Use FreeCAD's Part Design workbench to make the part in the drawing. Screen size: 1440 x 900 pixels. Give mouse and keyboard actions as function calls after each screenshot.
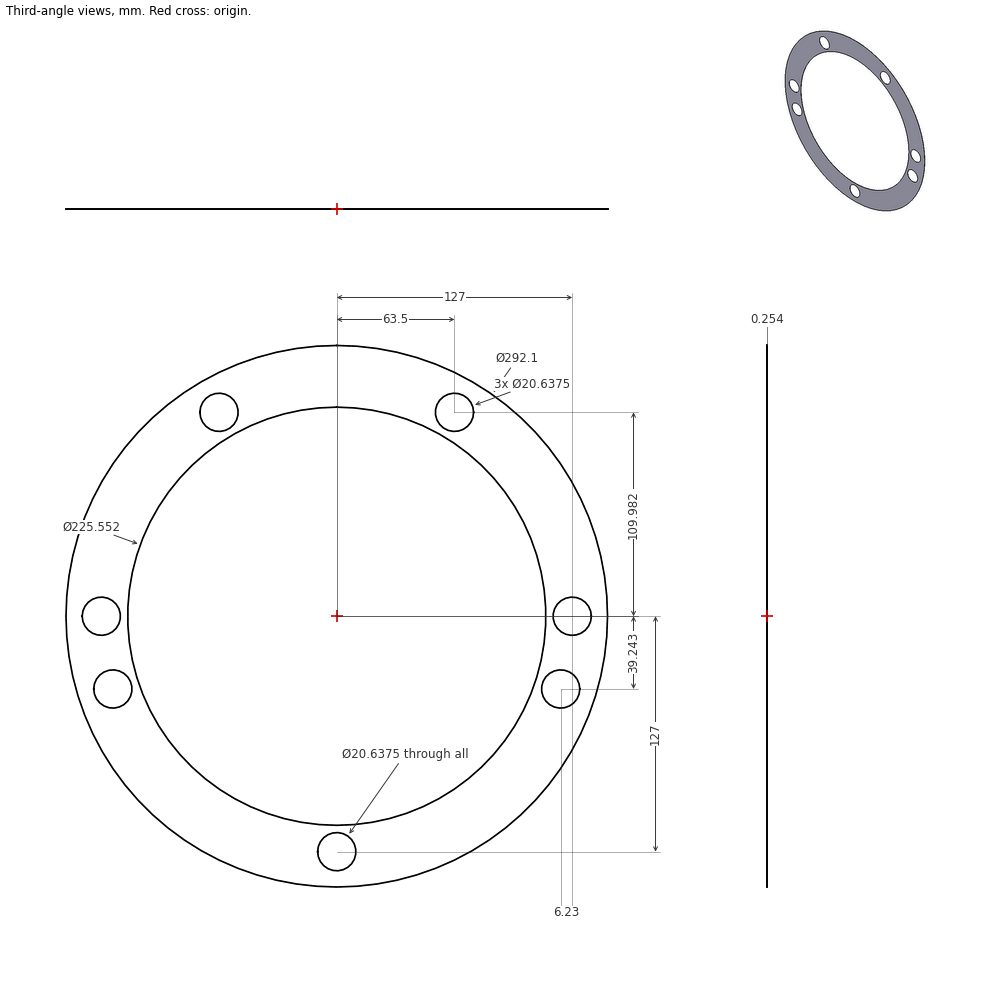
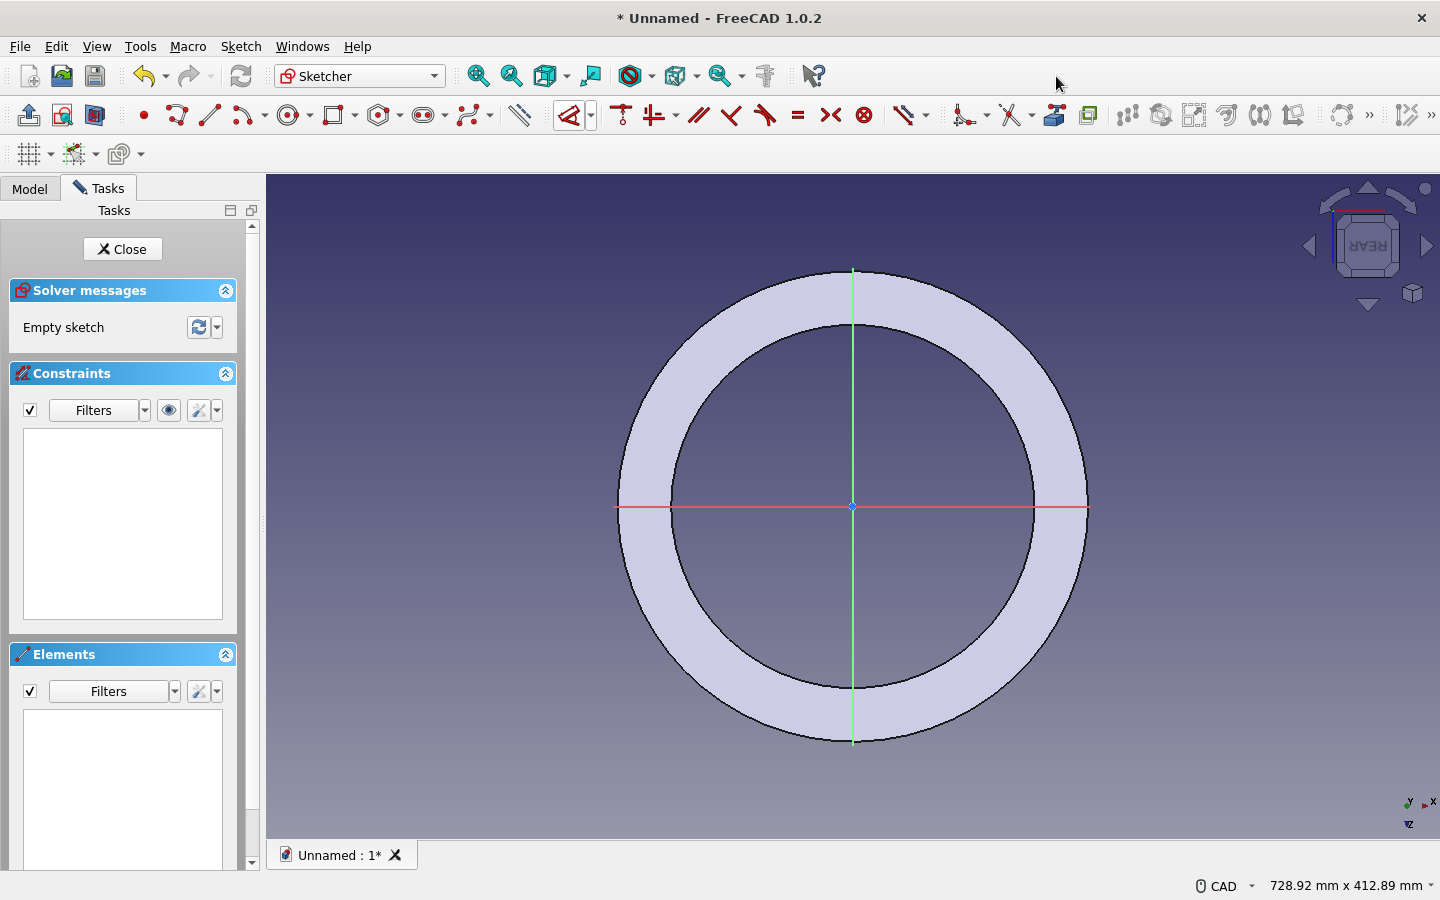
scroll(858, 286, up, 13)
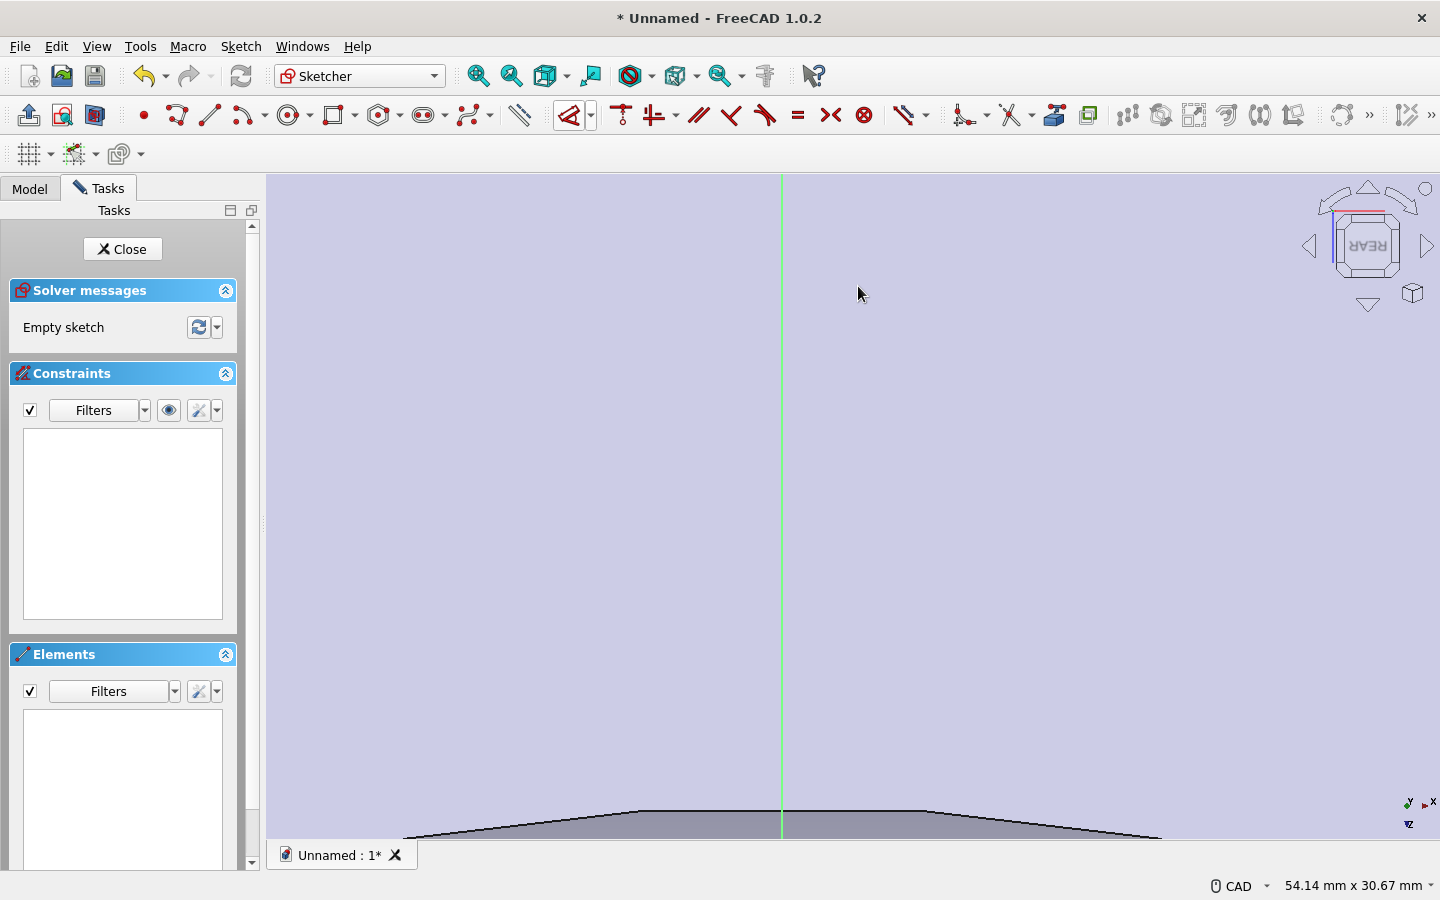
key(g)
key(c)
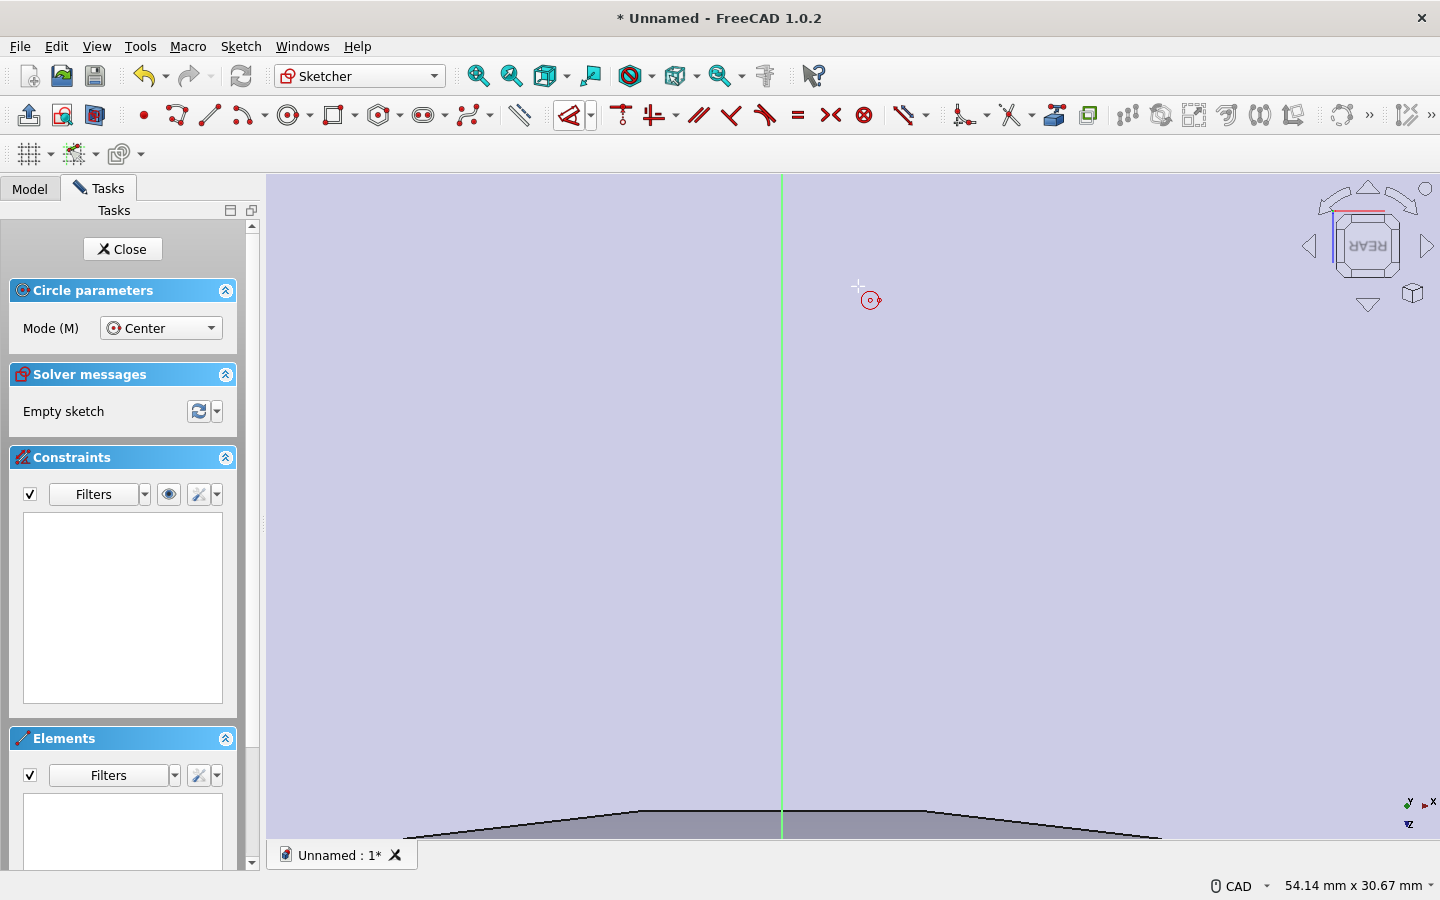
click(782, 499)
click(941, 340)
key(Escape)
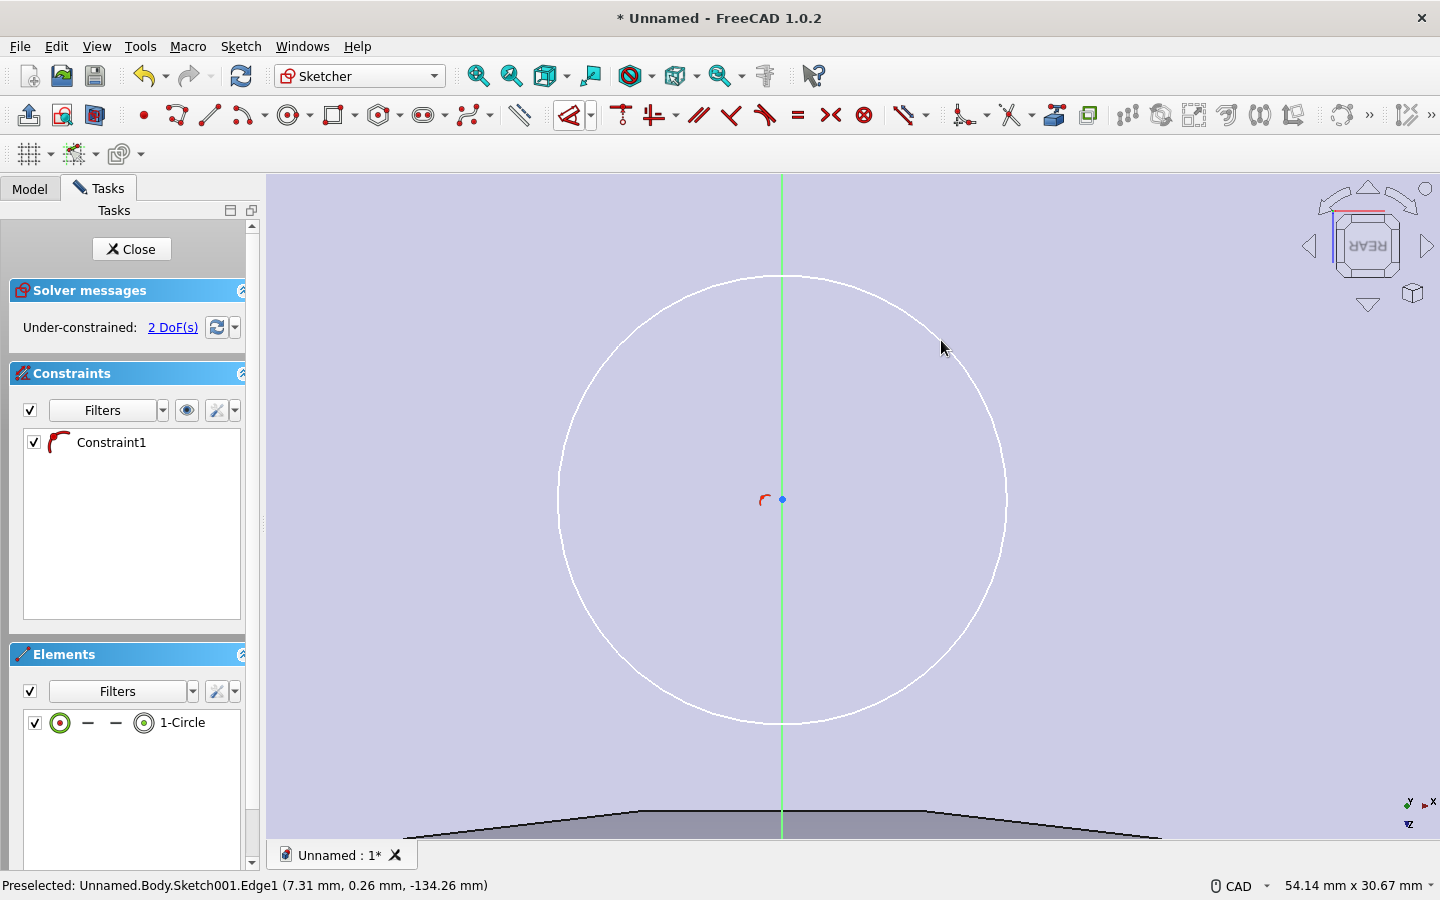
click(941, 341)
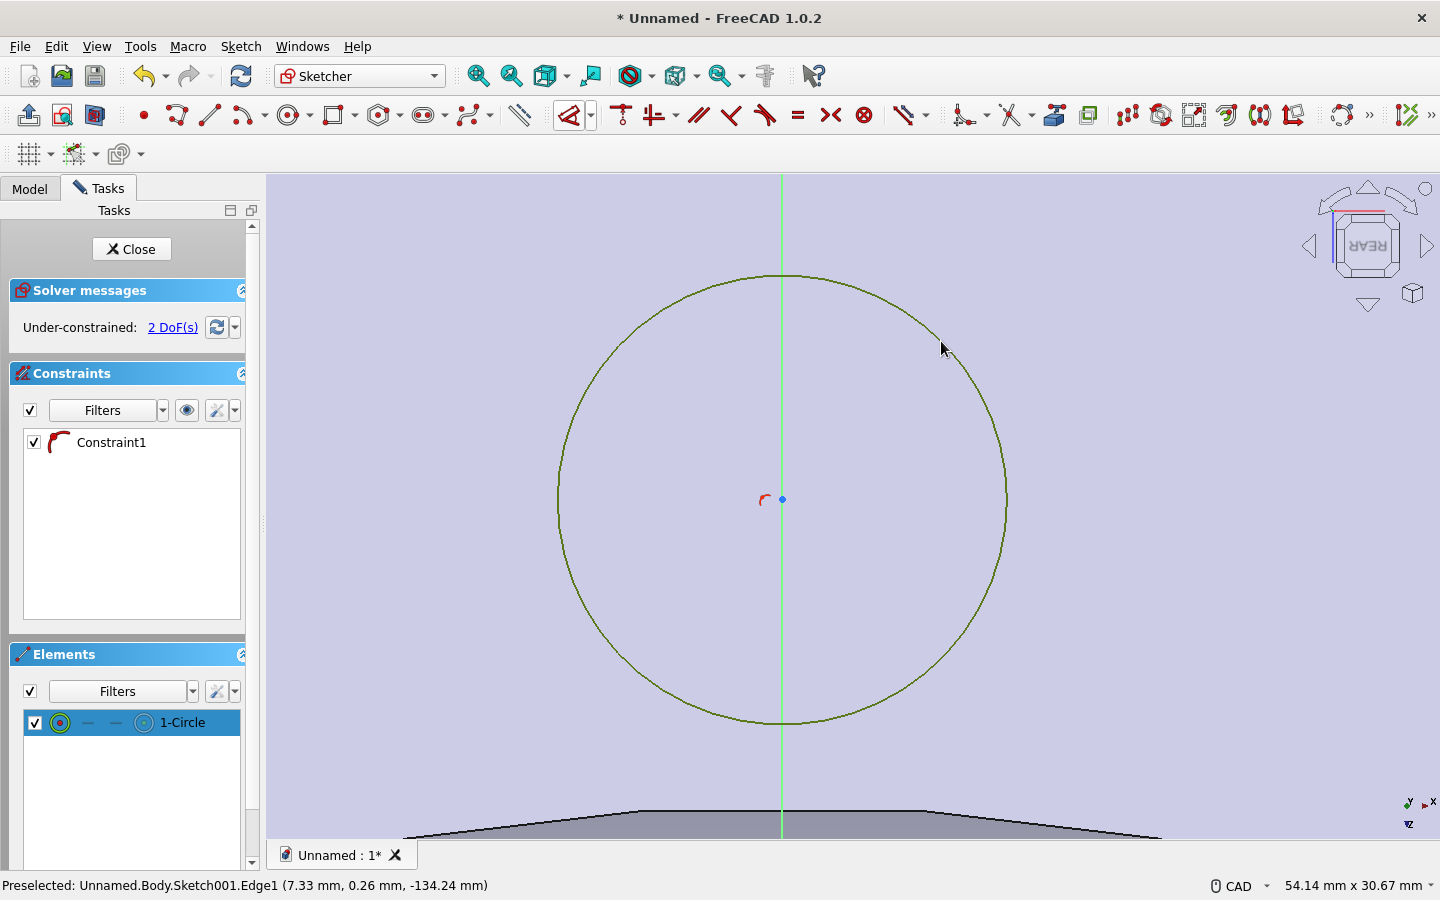
key(k)
key(o)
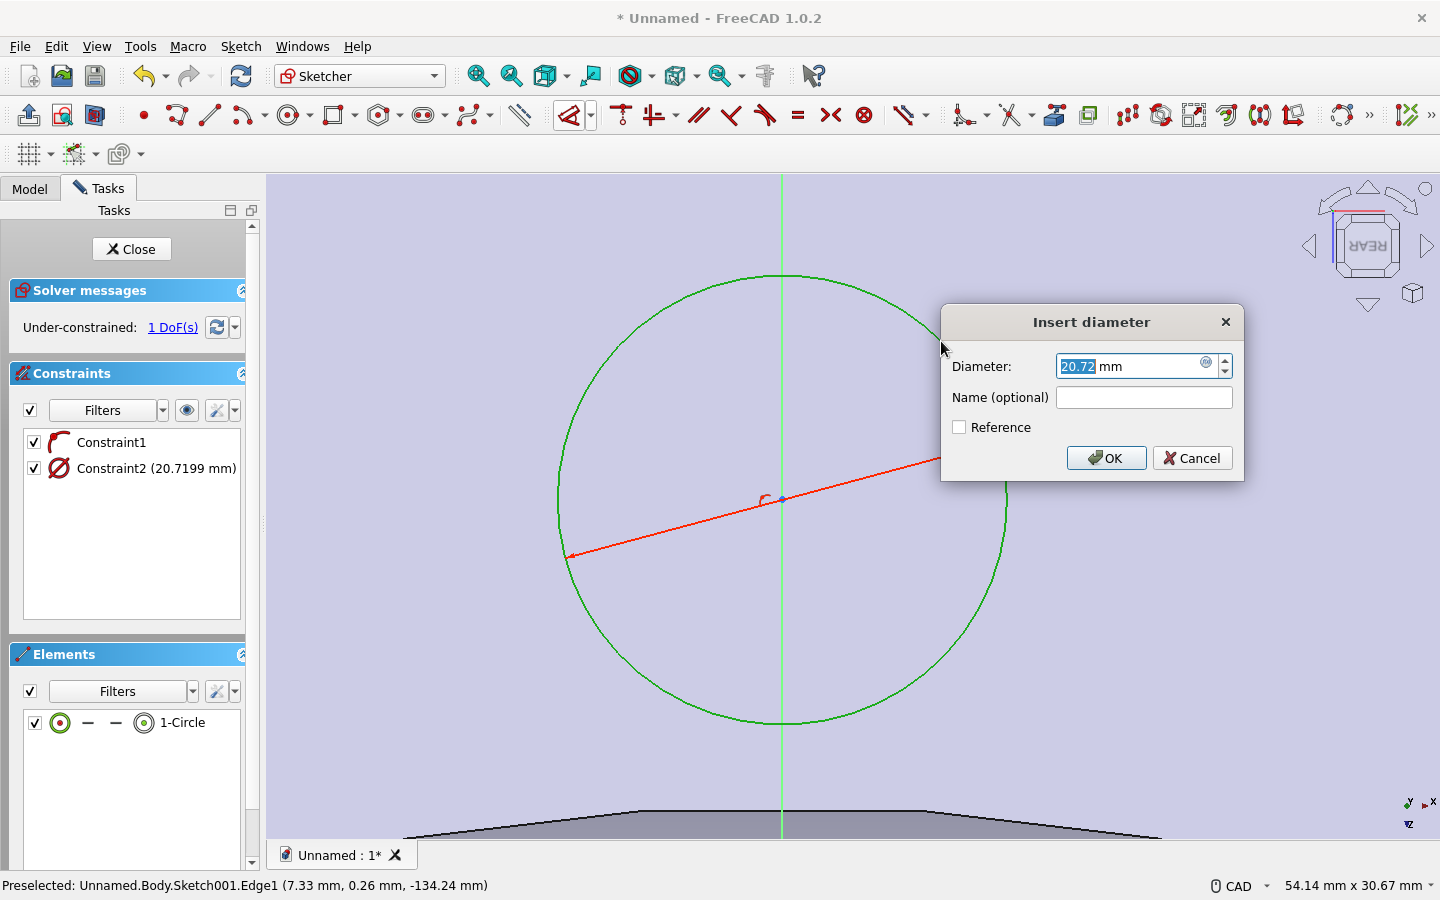
text(20.6375)
key(Return)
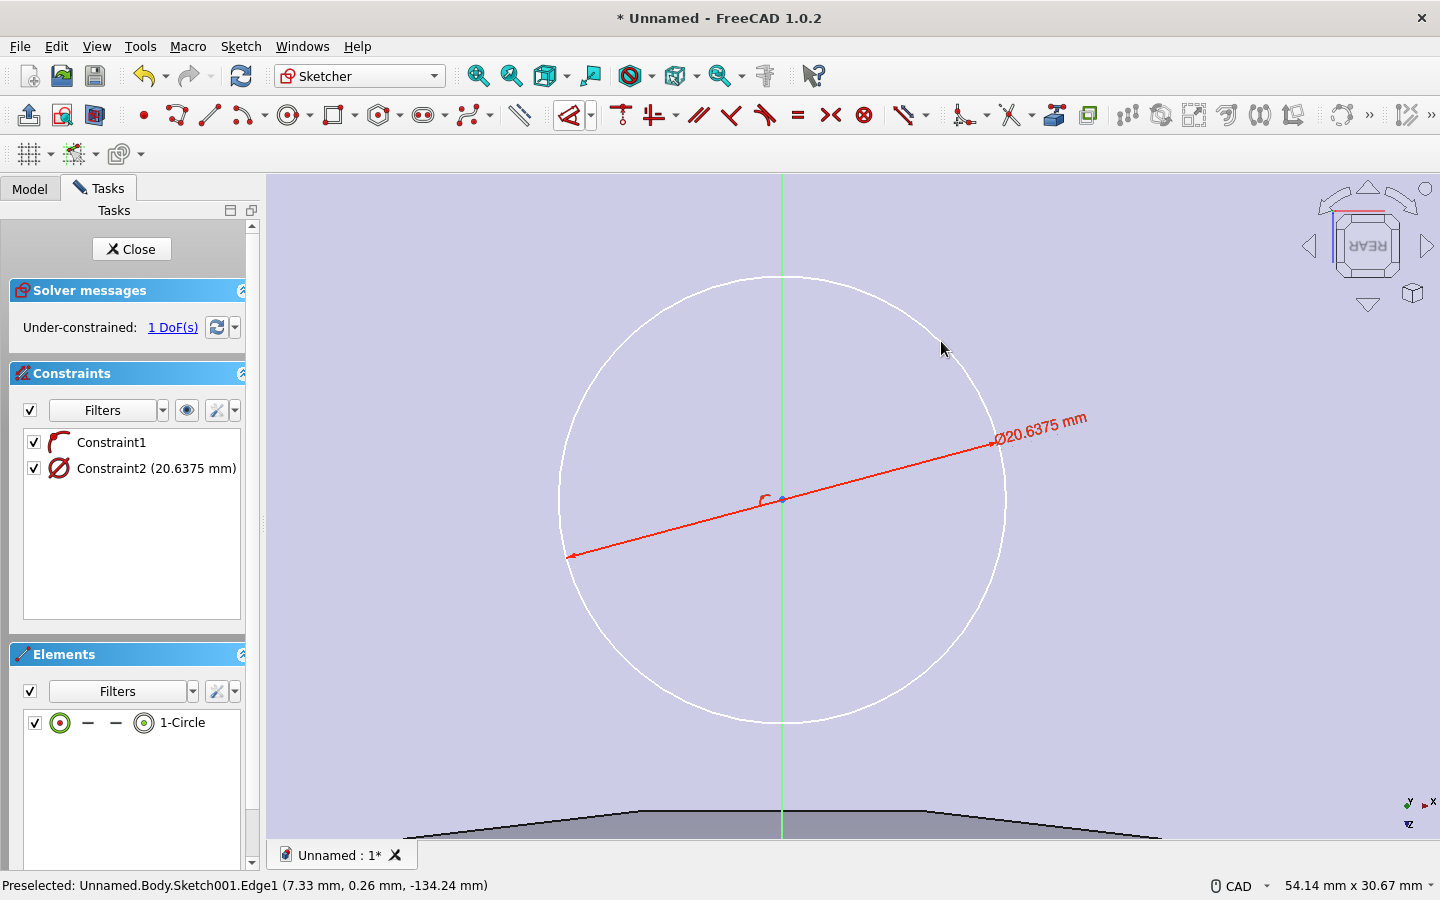
click(782, 500)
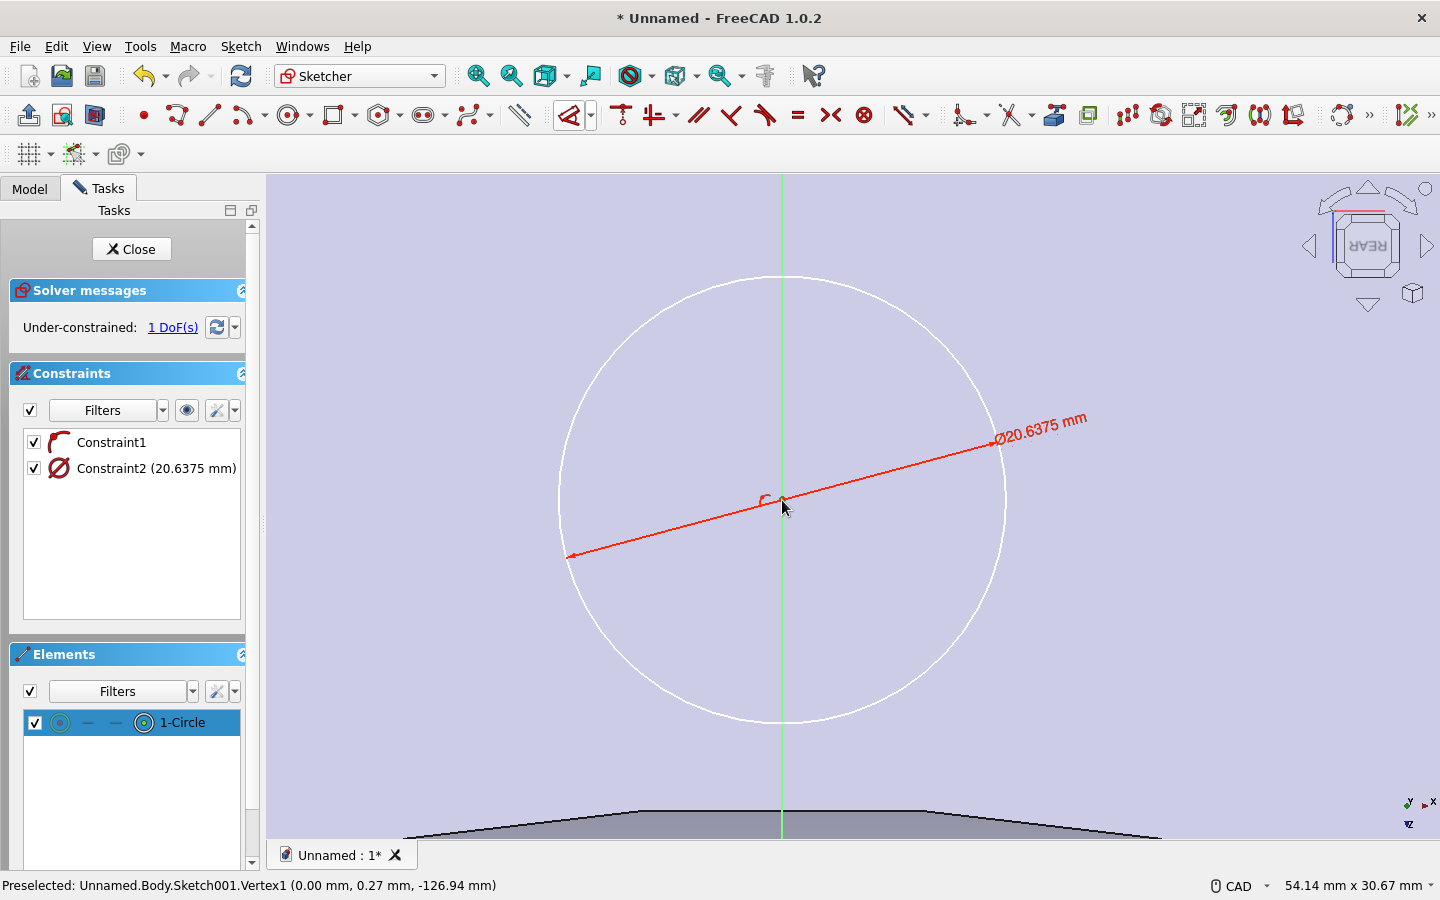
key(i)